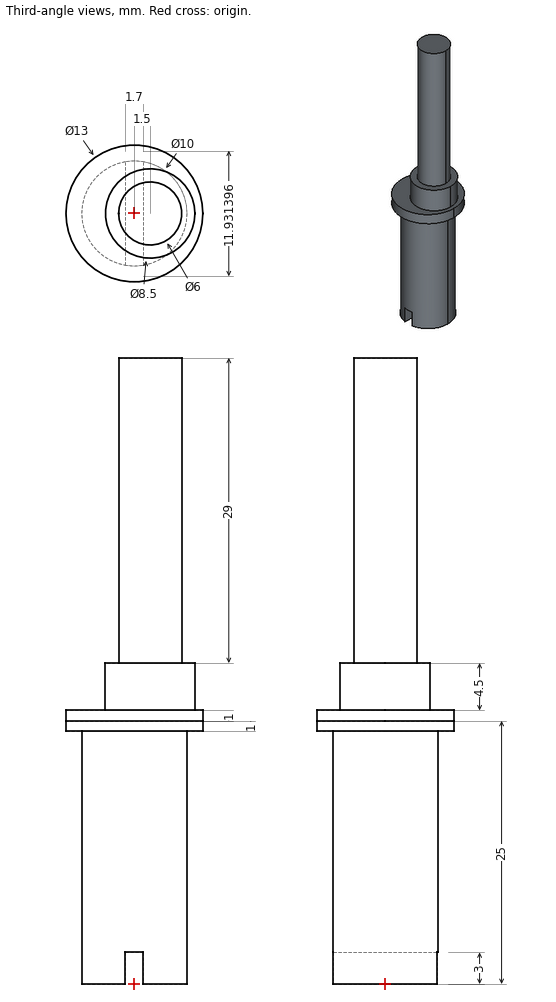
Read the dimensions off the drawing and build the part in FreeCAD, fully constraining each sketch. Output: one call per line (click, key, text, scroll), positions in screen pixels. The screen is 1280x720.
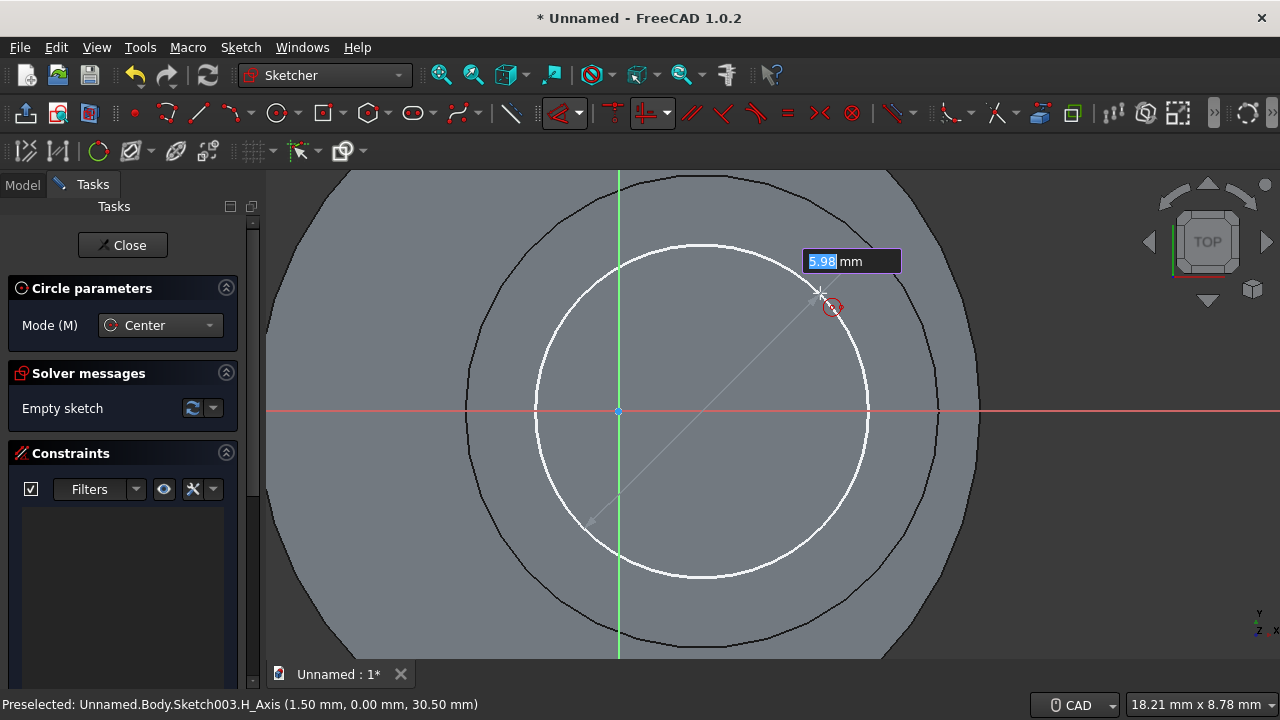
text(6)
key(Return)
key(Escape)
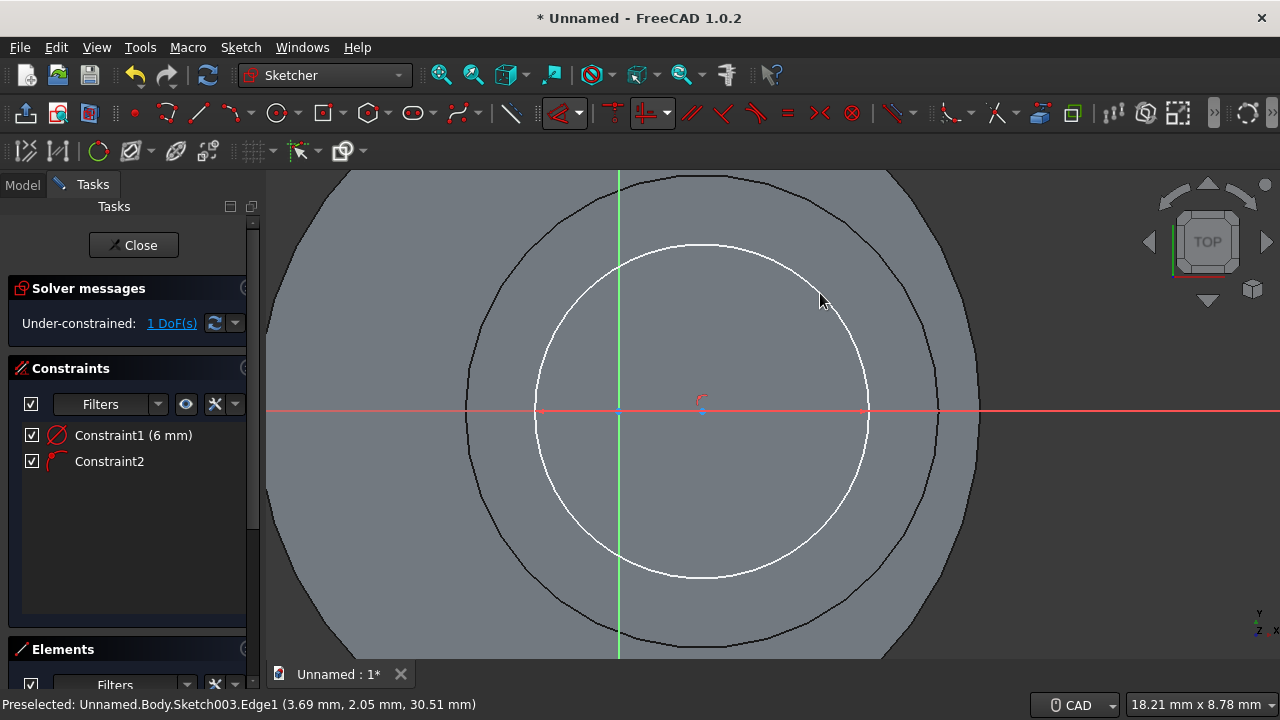
click(702, 411)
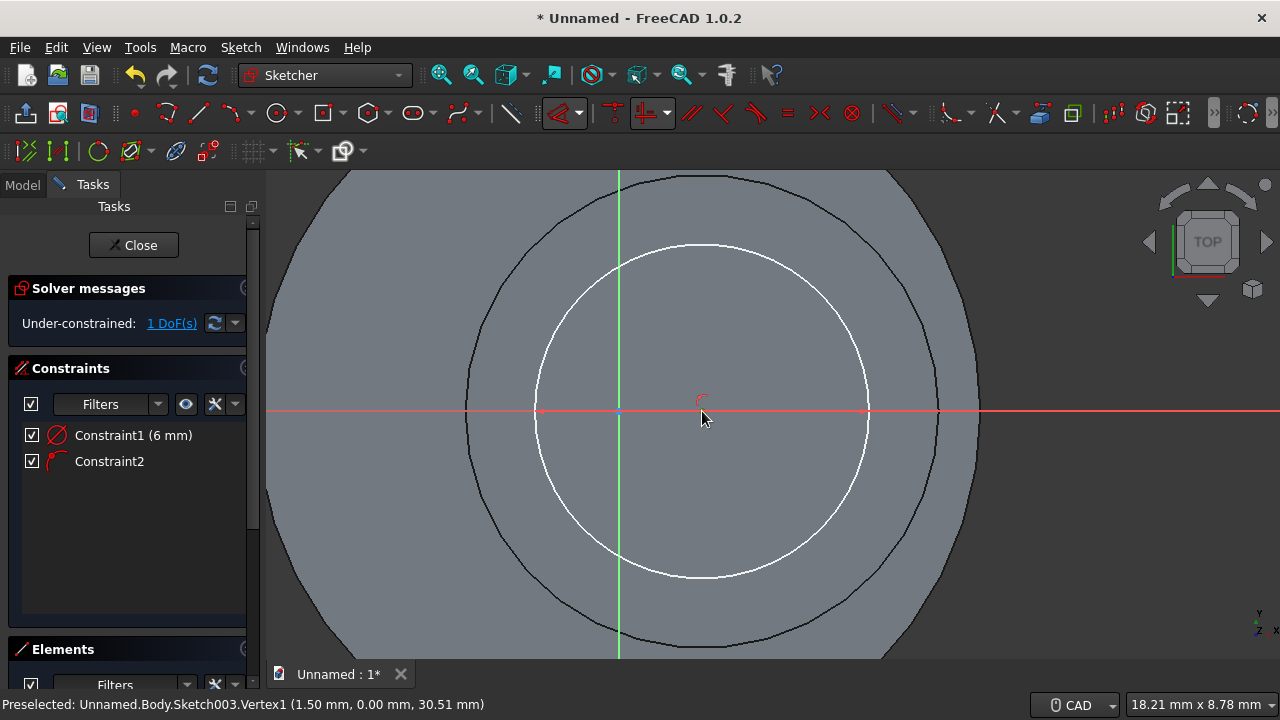
click(582, 114)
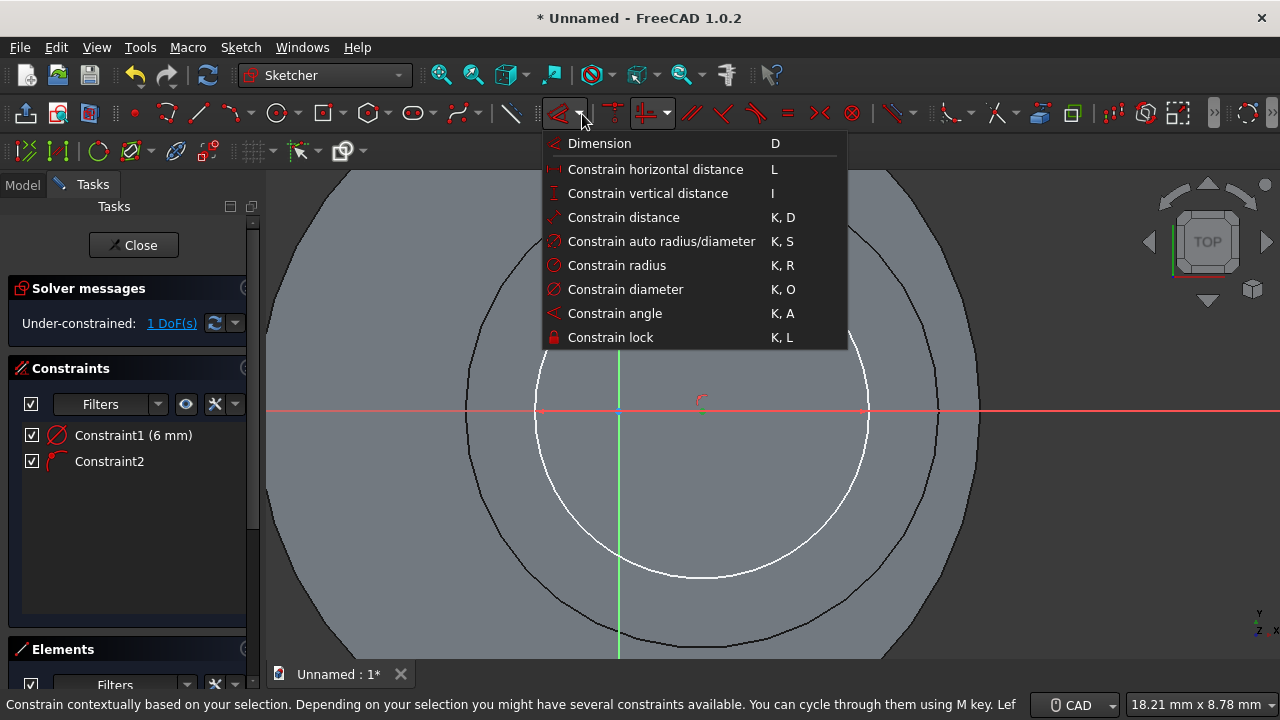
click(695, 169)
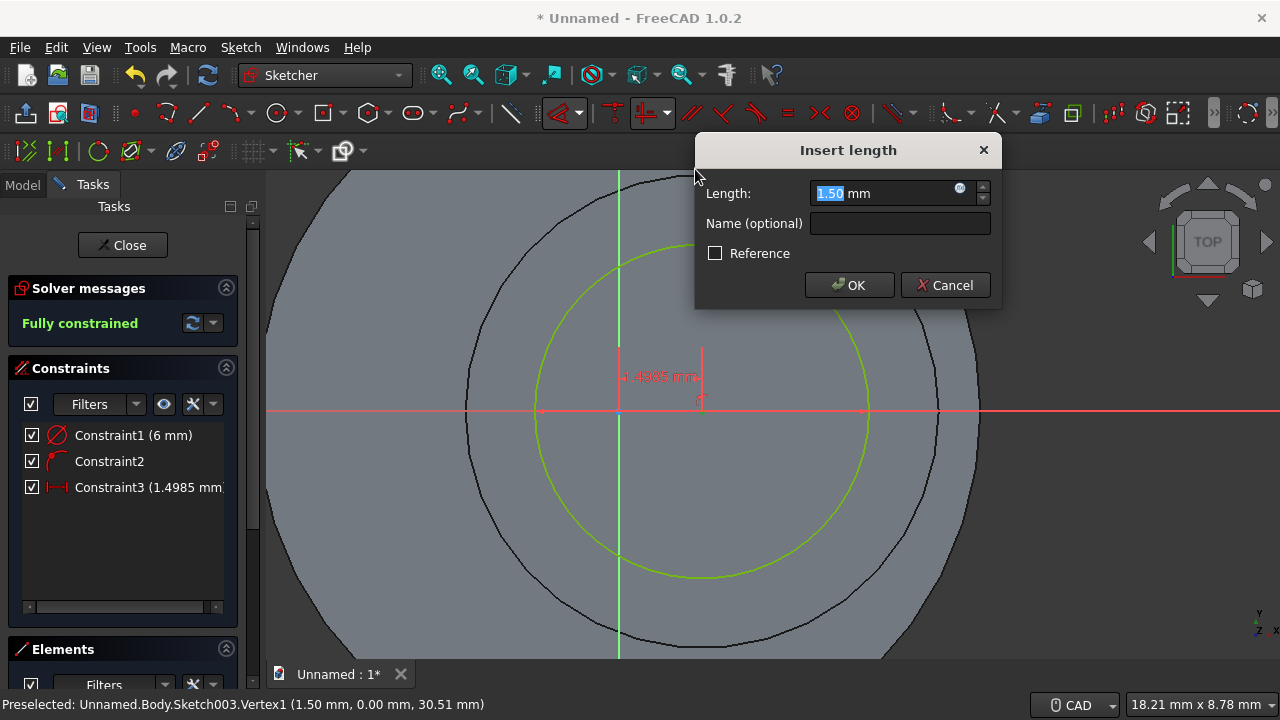
text(1.5)
key(Return)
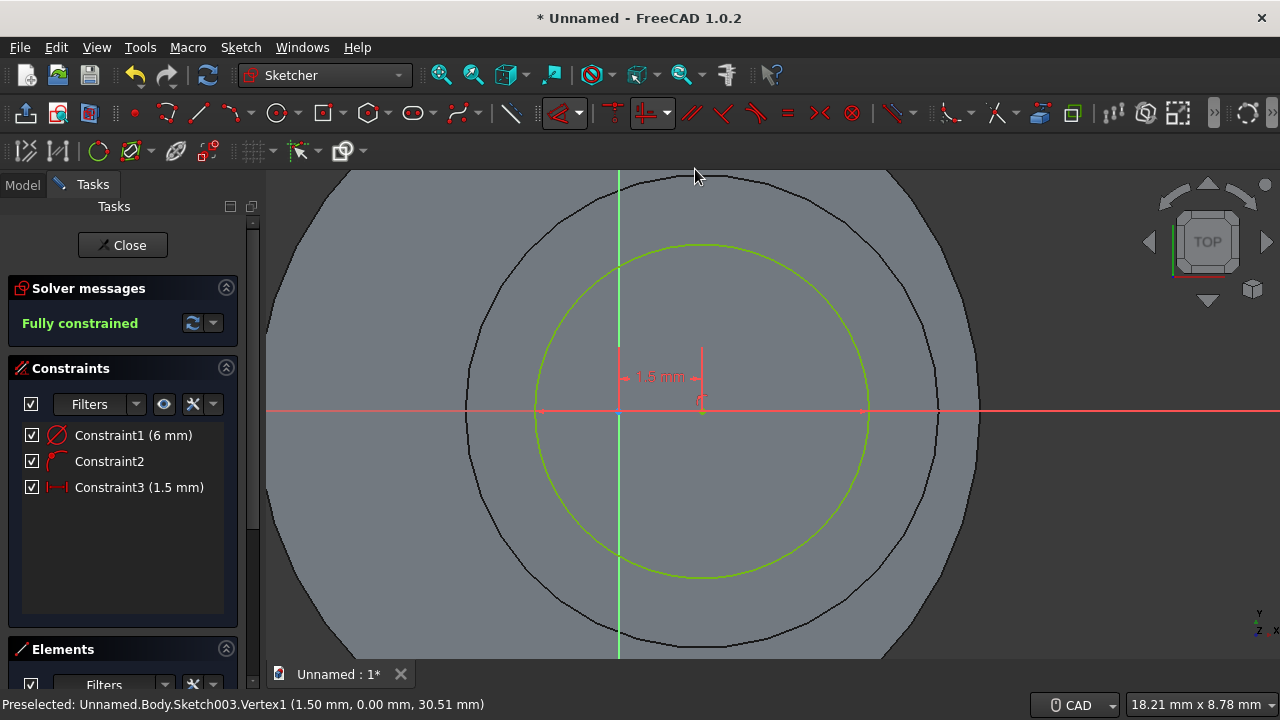
click(123, 245)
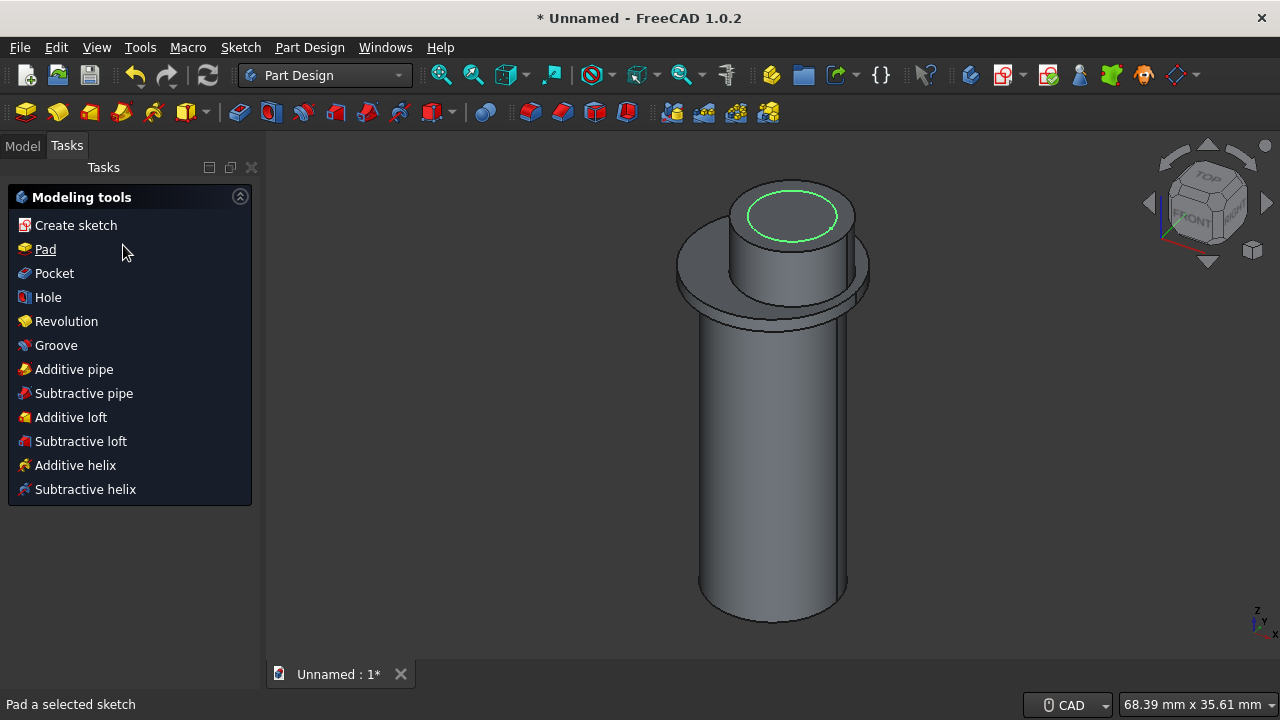
click(26, 112)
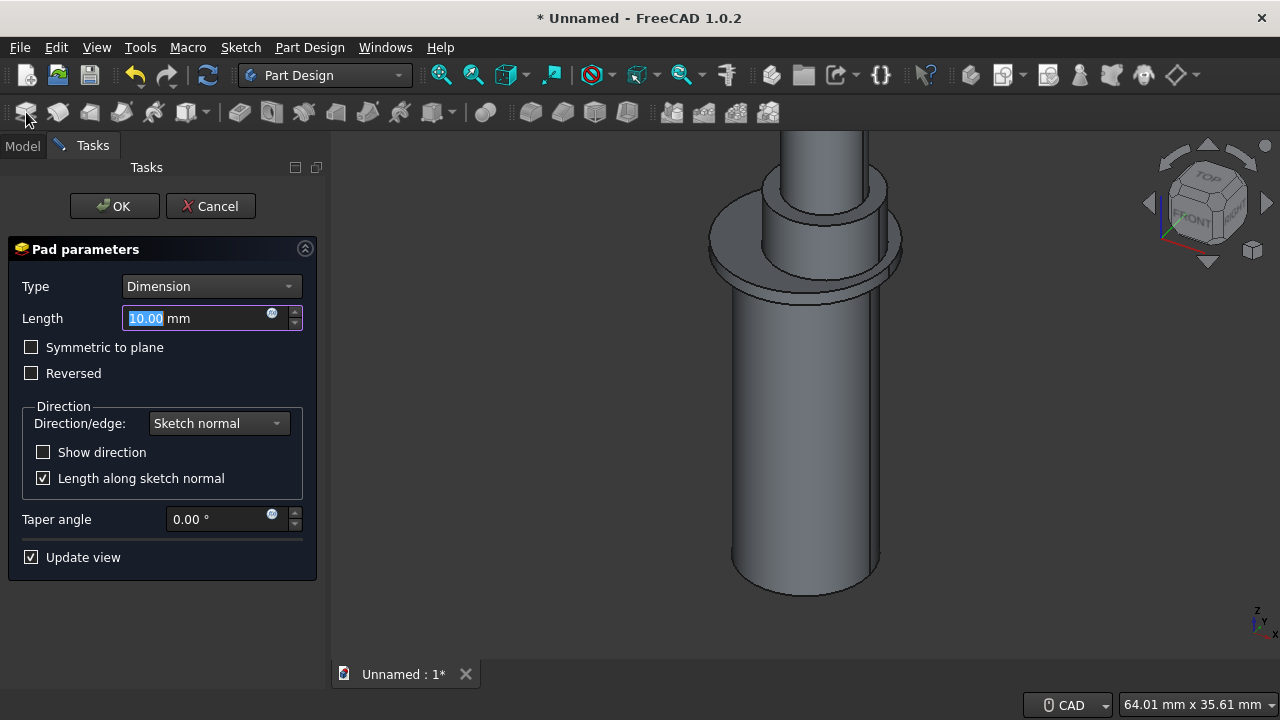
text(29)
key(Tab)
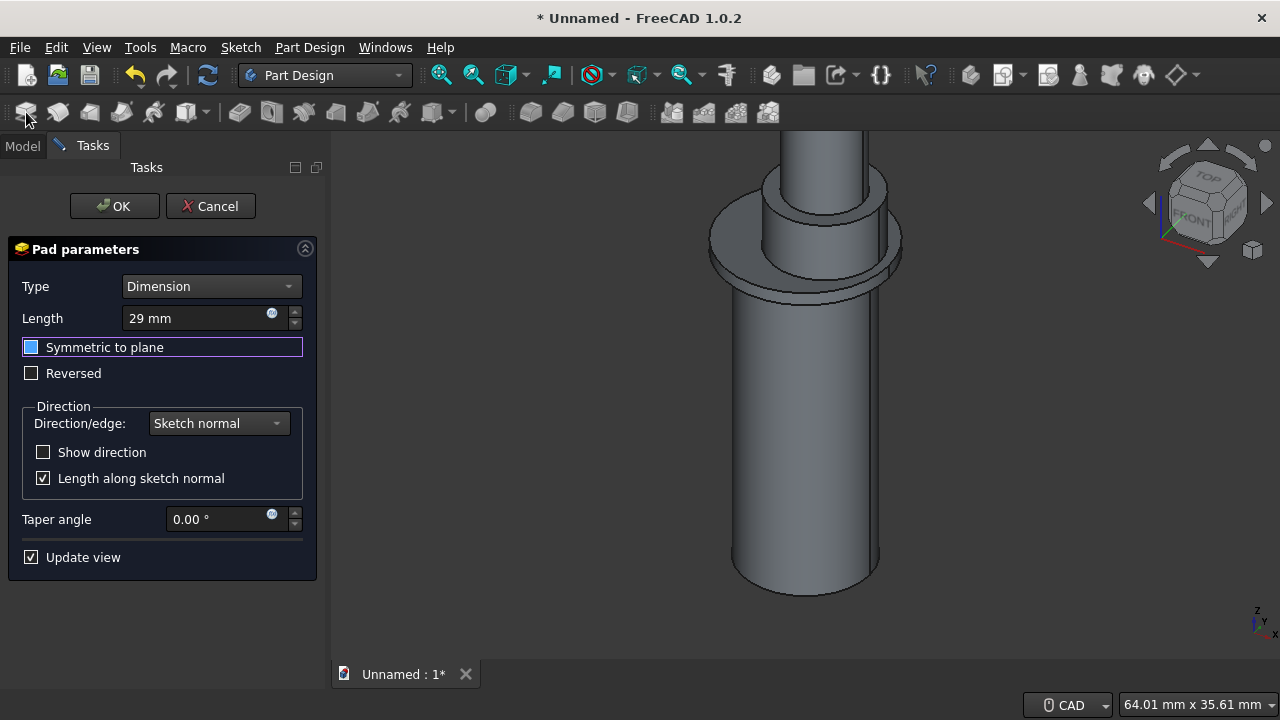
click(115, 206)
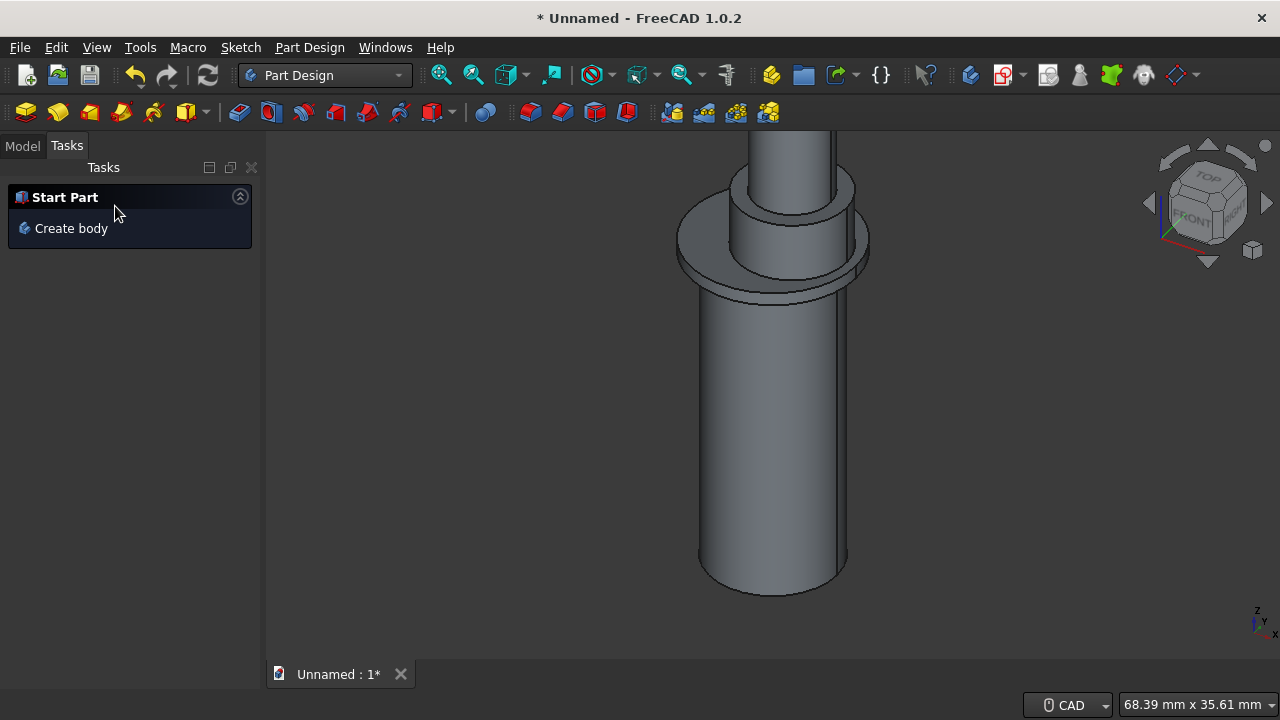
click(442, 76)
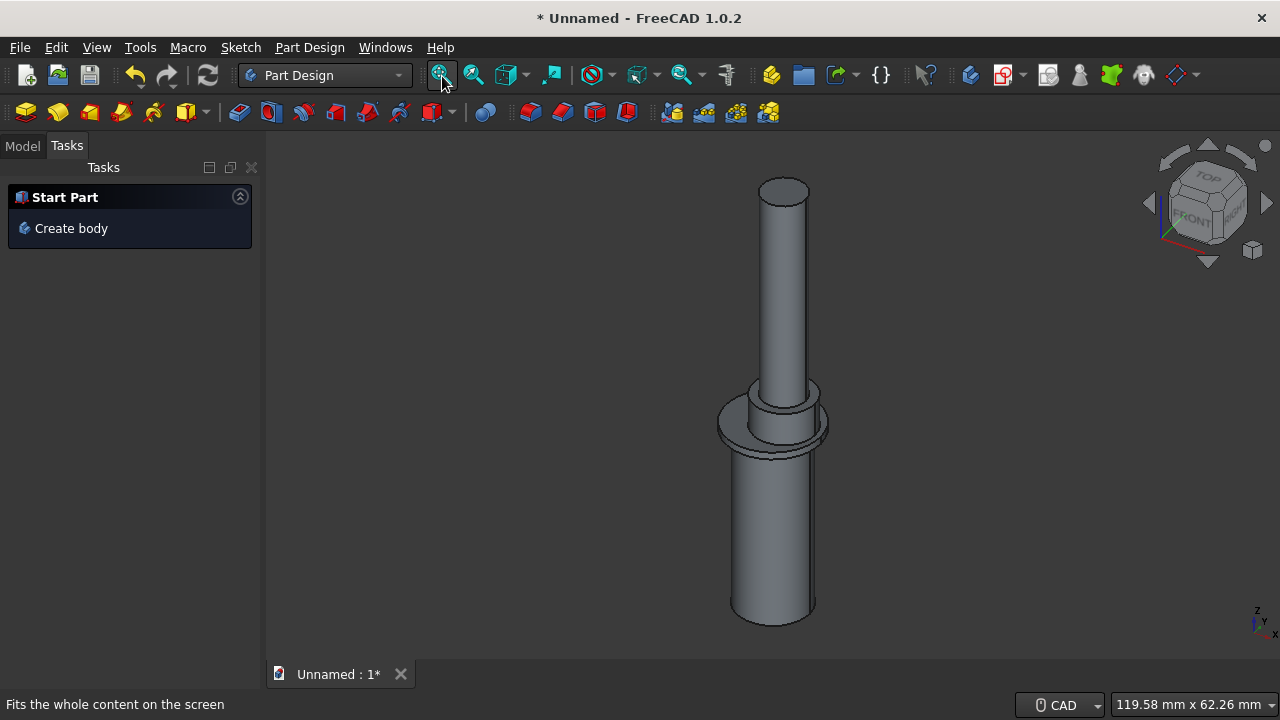
key(5)